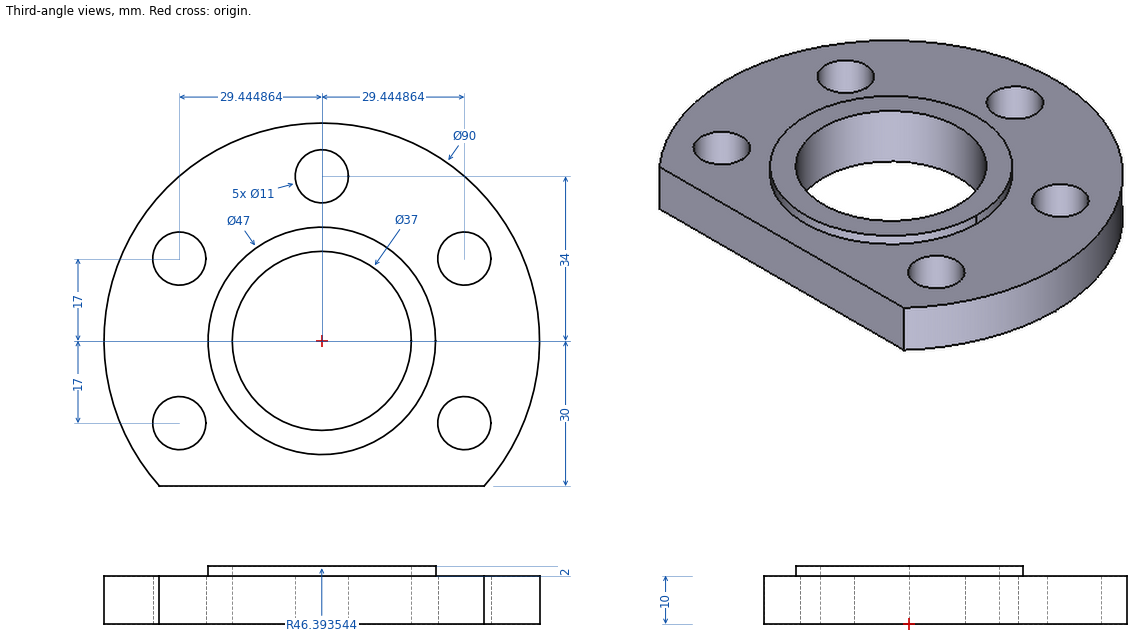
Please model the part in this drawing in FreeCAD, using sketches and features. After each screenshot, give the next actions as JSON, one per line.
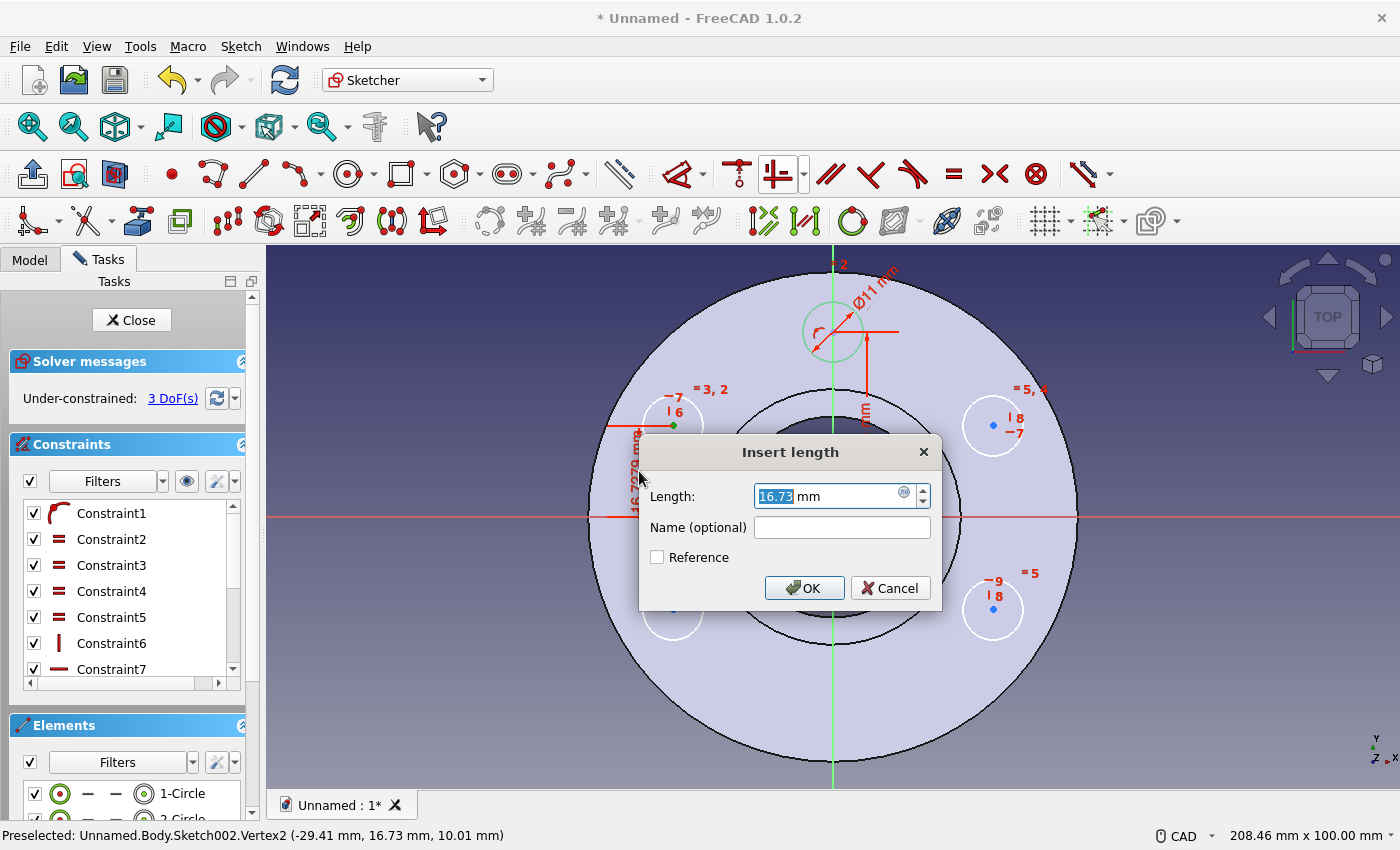
{"action": "type", "text": "17"}
{"action": "key", "text": "Return"}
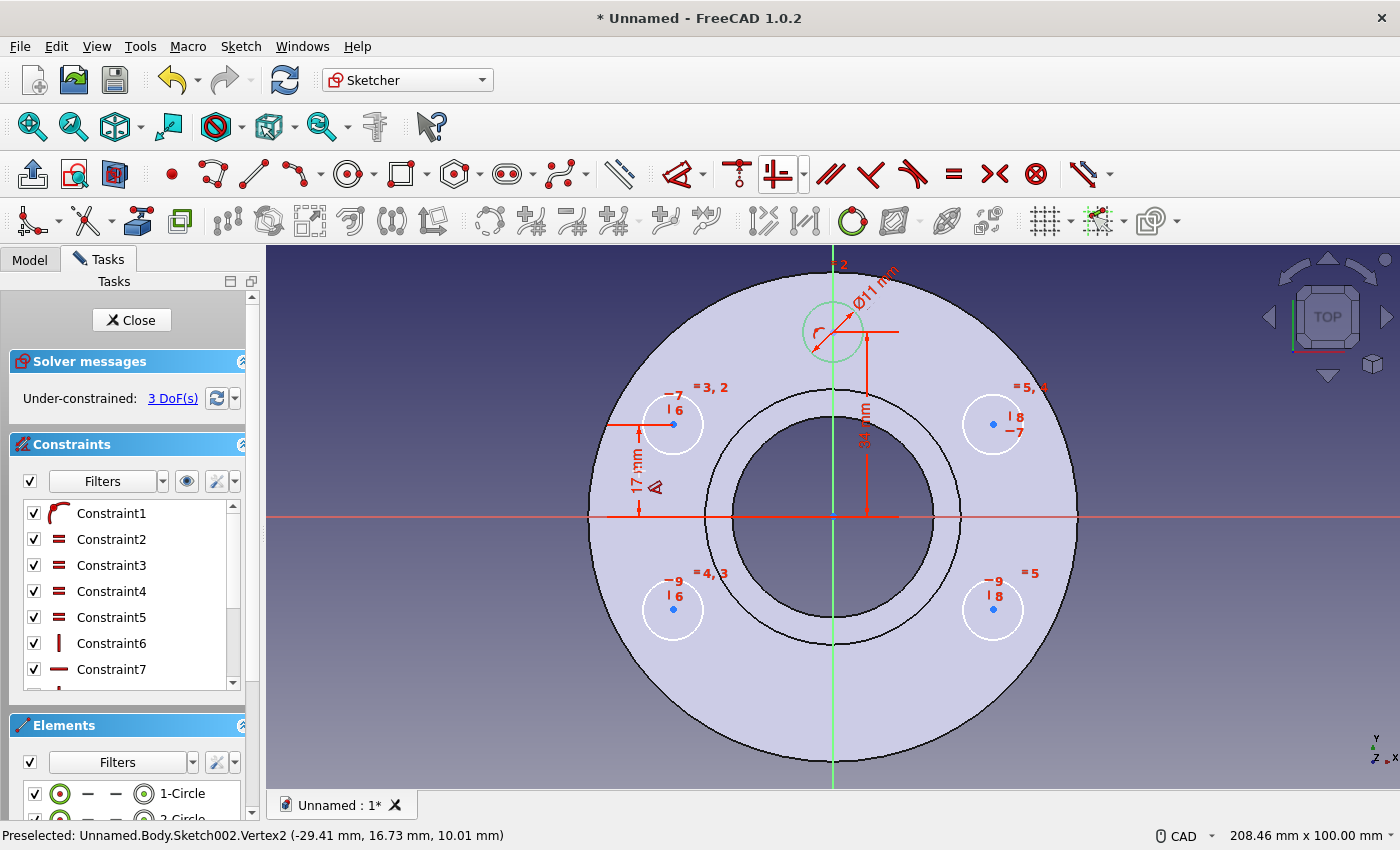
{"action": "left_click", "coordinate": [673, 610]}
{"action": "left_click", "coordinate": [639, 564]}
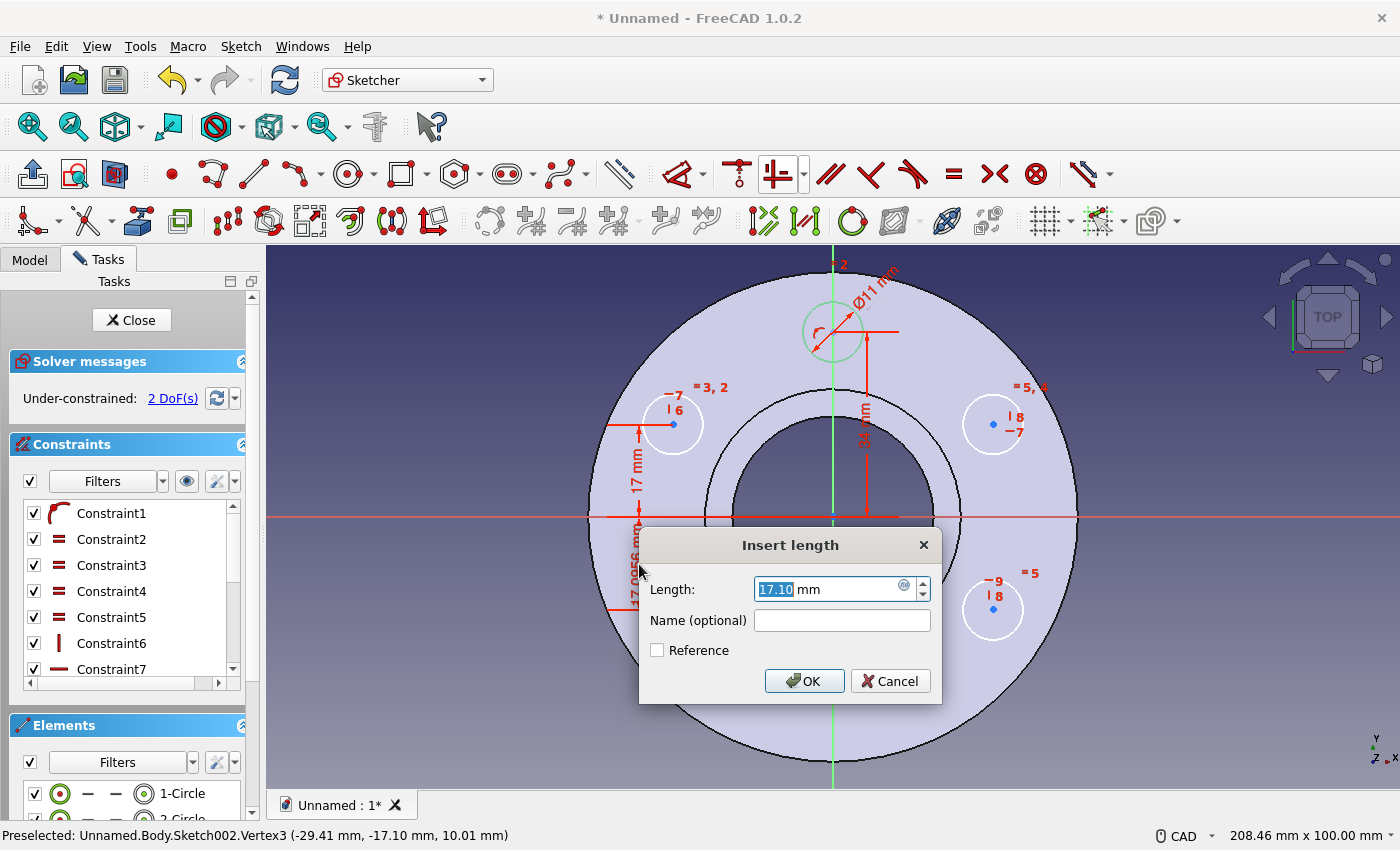
{"action": "type", "text": "17"}
{"action": "key", "text": "Return"}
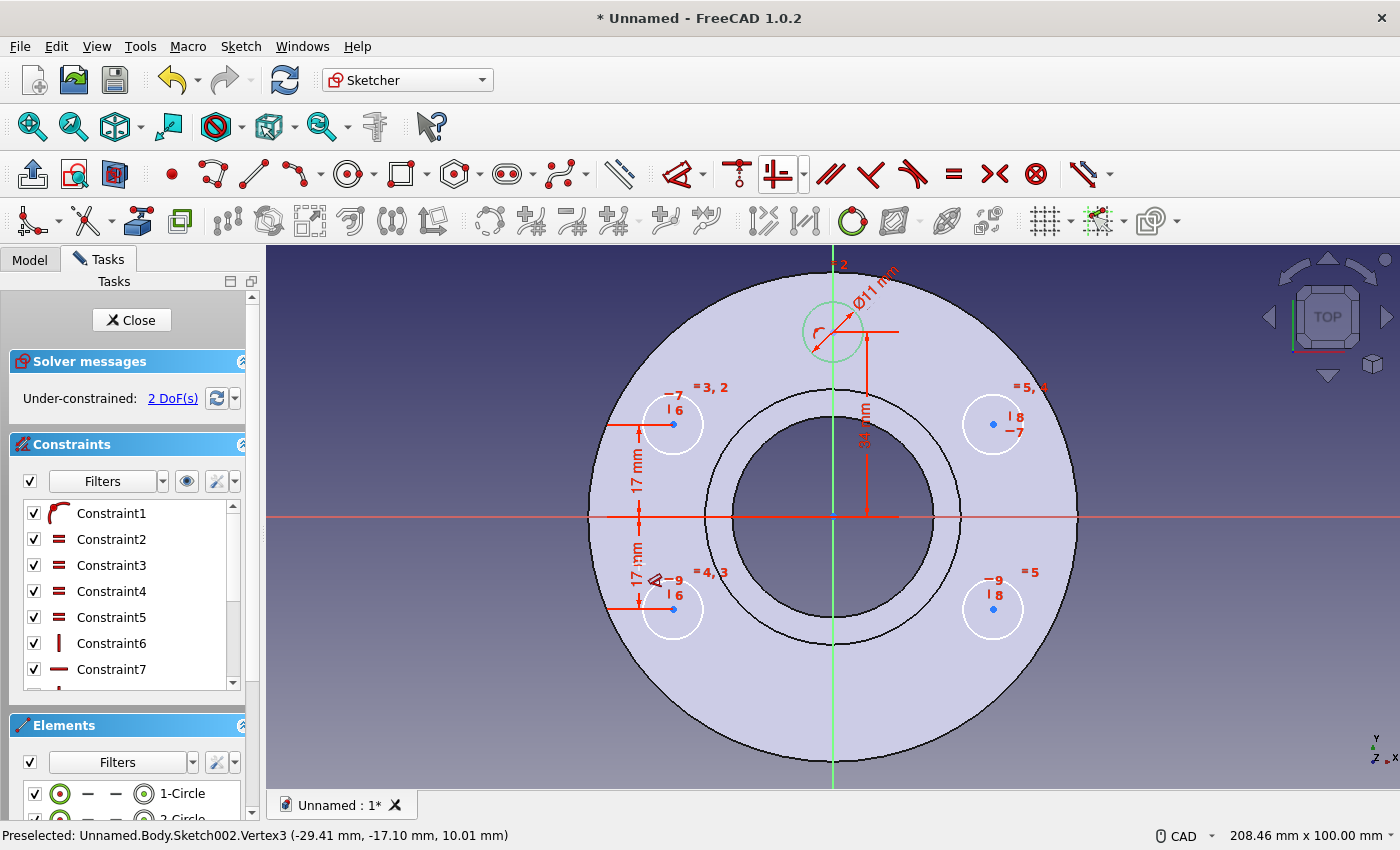
{"action": "left_click", "coordinate": [673, 425]}
{"action": "left_click", "coordinate": [753, 551]}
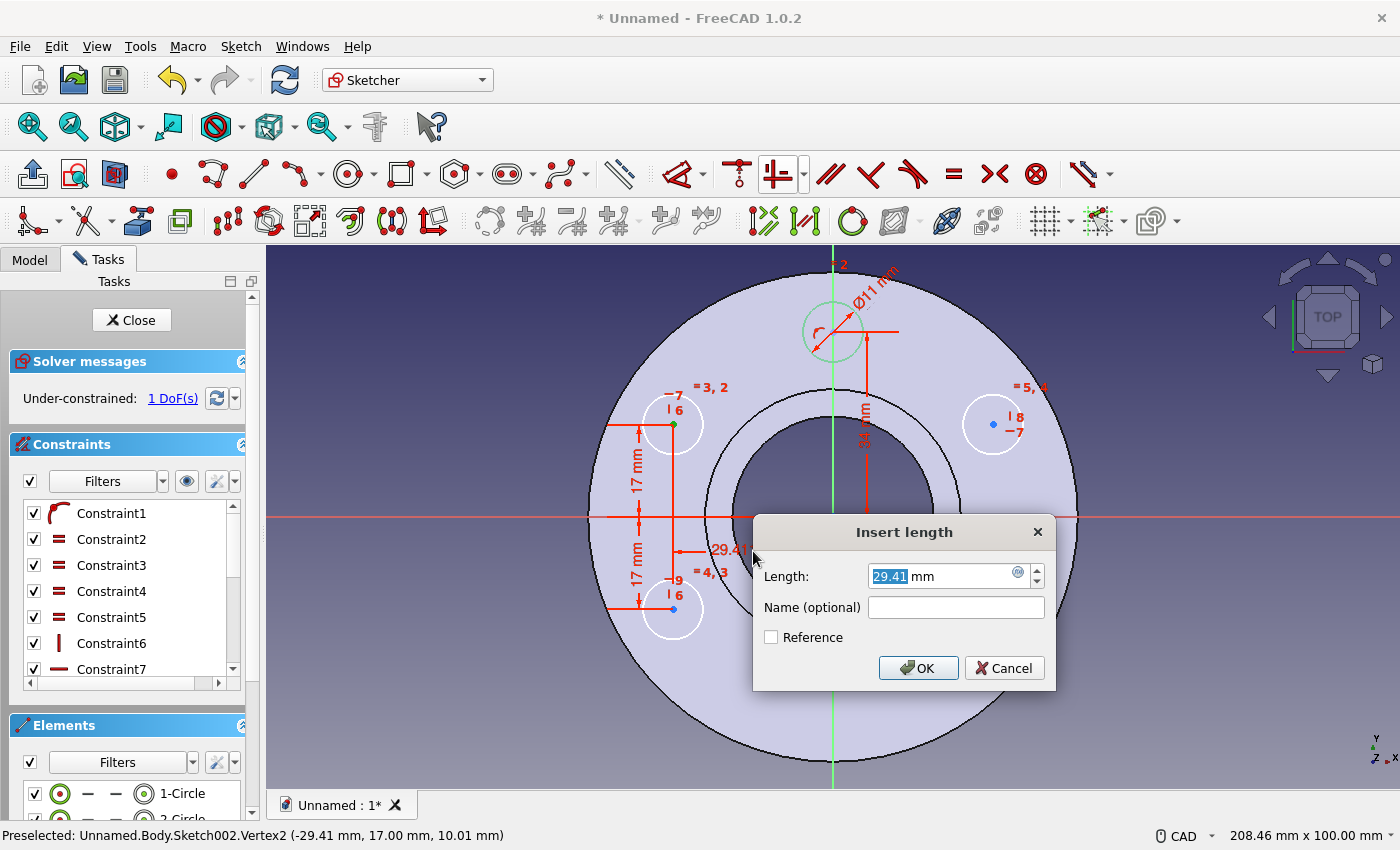
{"action": "type", "text": "29.444864"}
{"action": "key", "text": "Return"}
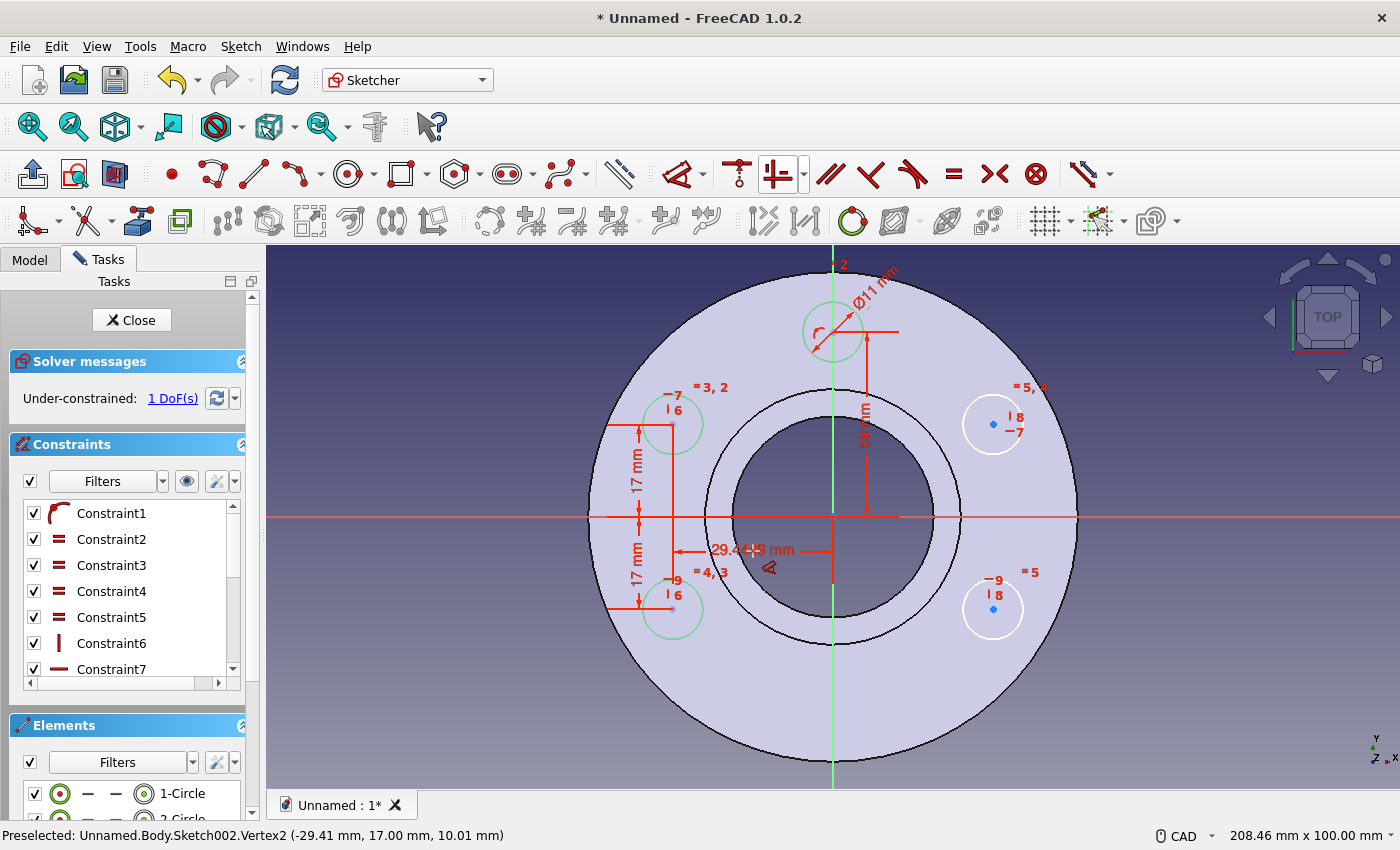
{"action": "left_click", "coordinate": [993, 425]}
{"action": "left_click", "coordinate": [913, 551]}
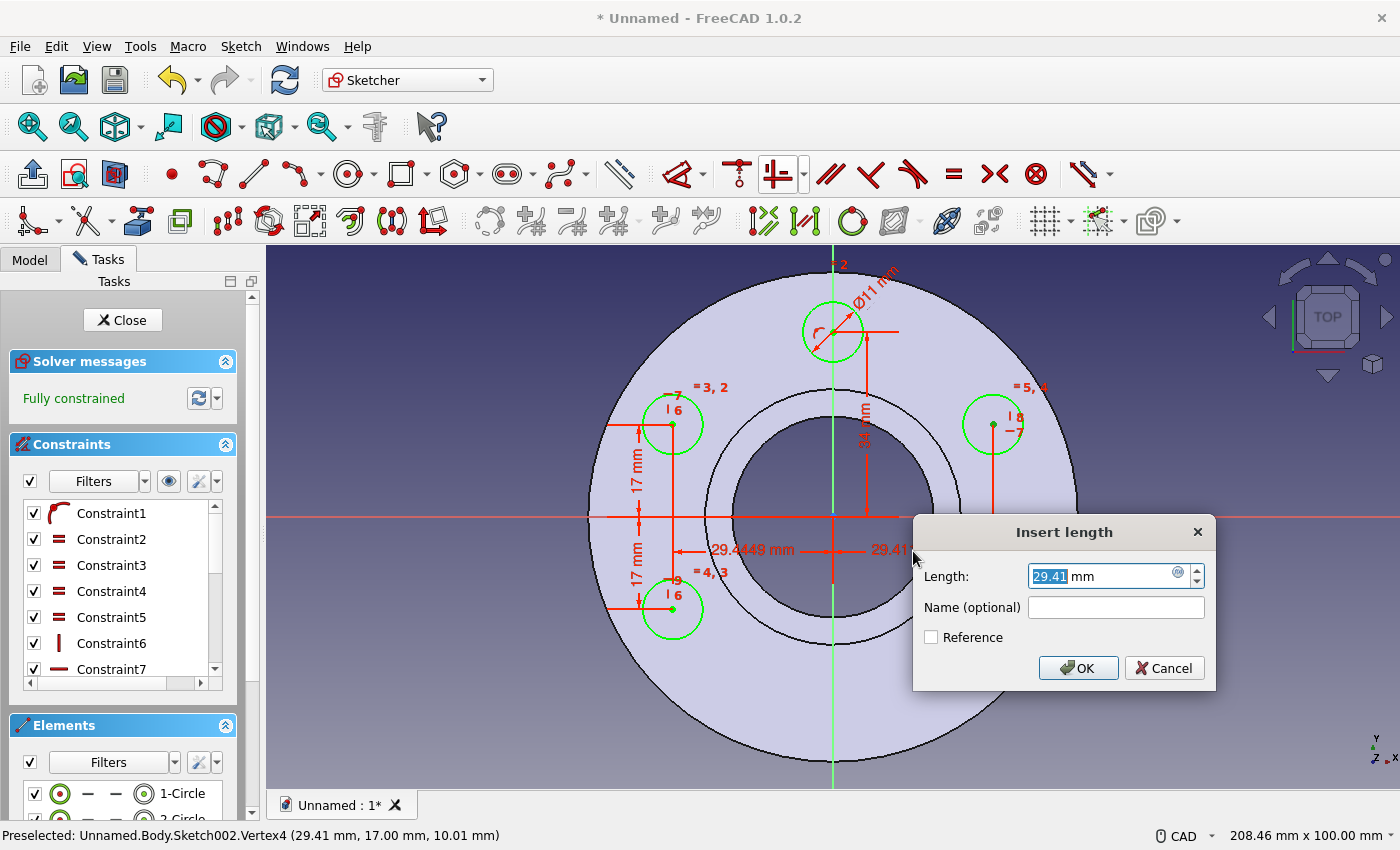
{"action": "type", "text": "29.444864"}
{"action": "key", "text": "Return"}
{"action": "key", "text": "Escape"}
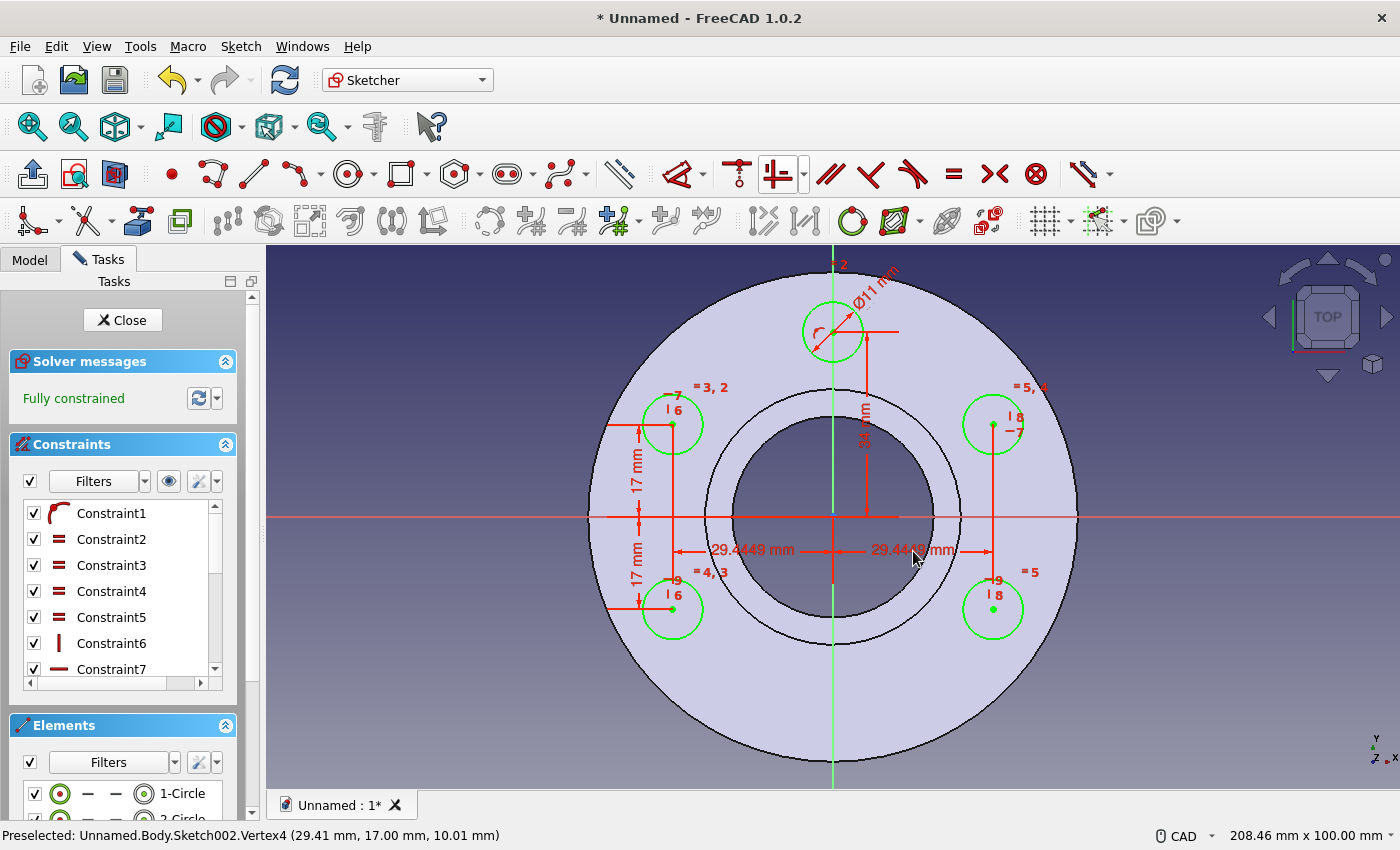
{"action": "left_click", "coordinate": [123, 320]}